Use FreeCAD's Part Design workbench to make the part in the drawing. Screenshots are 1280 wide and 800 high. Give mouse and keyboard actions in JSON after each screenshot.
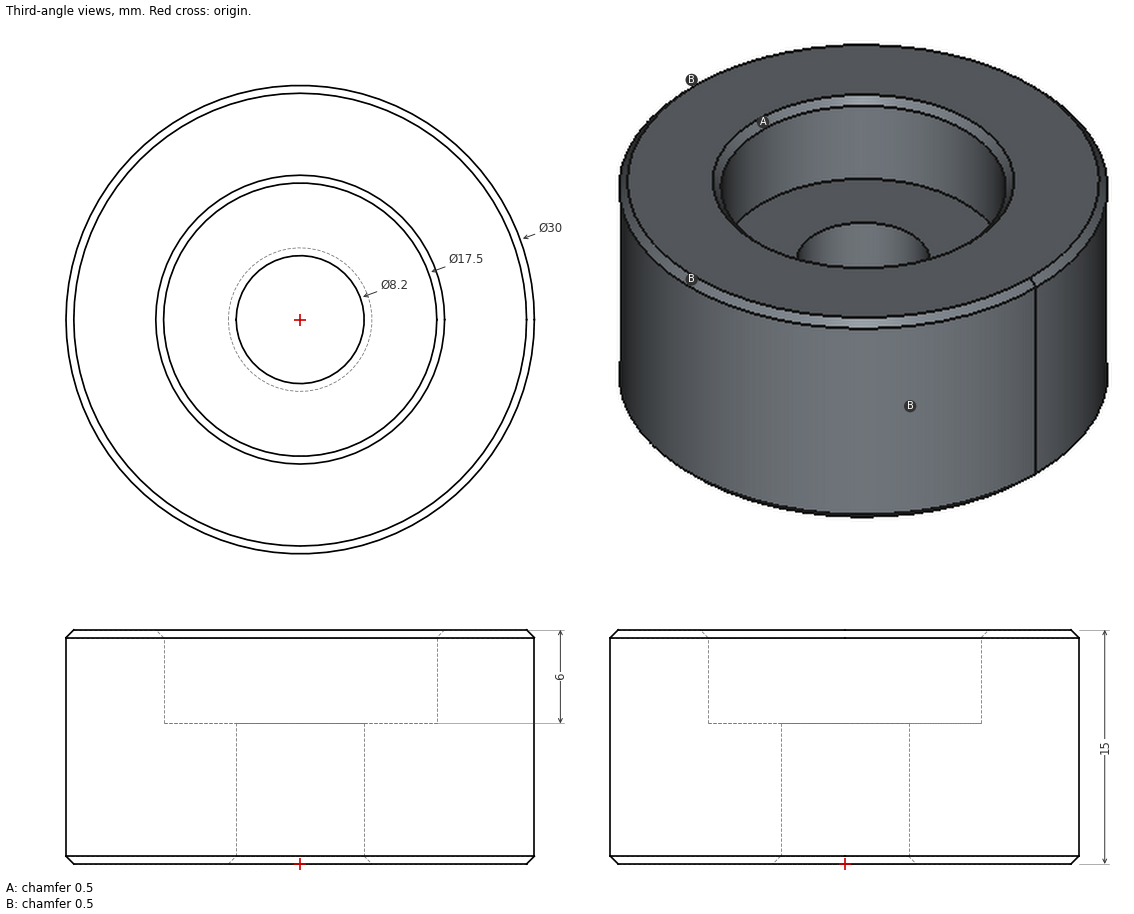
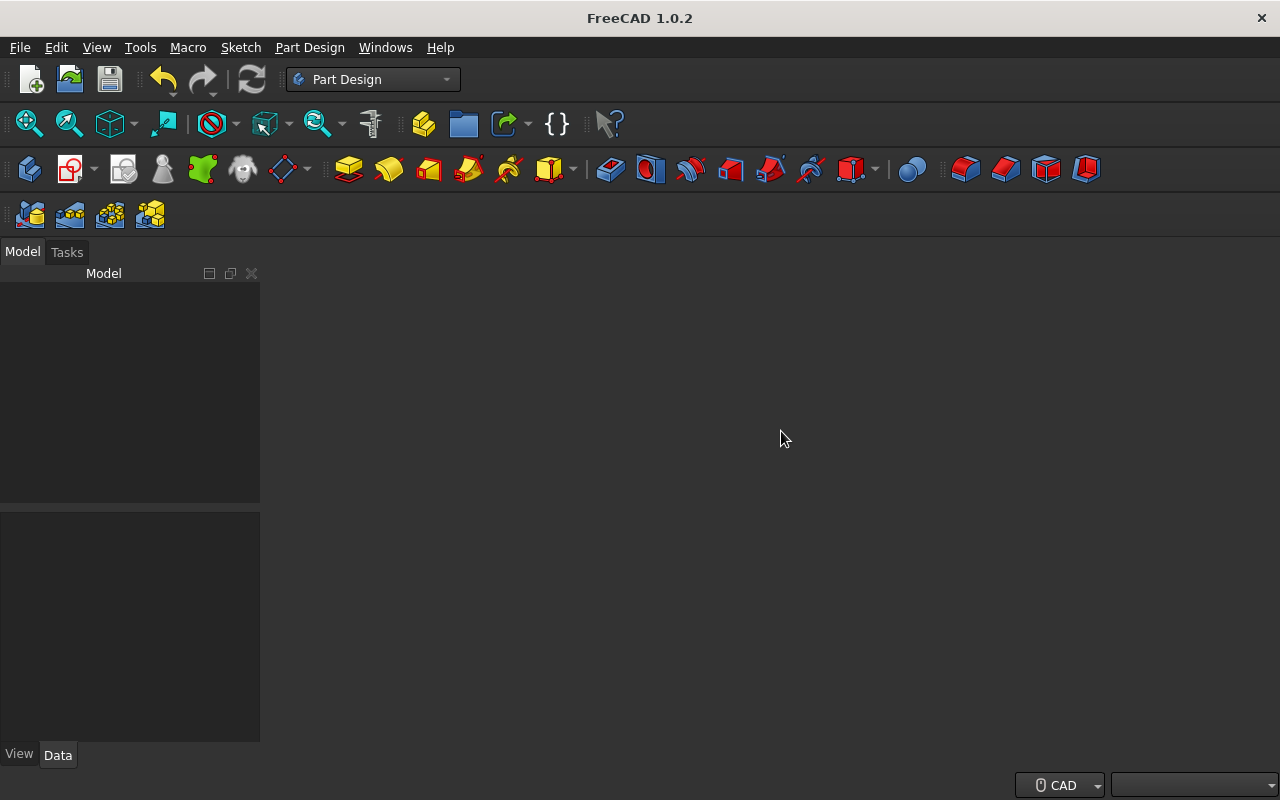
{"action": "key", "text": "ctrl+n"}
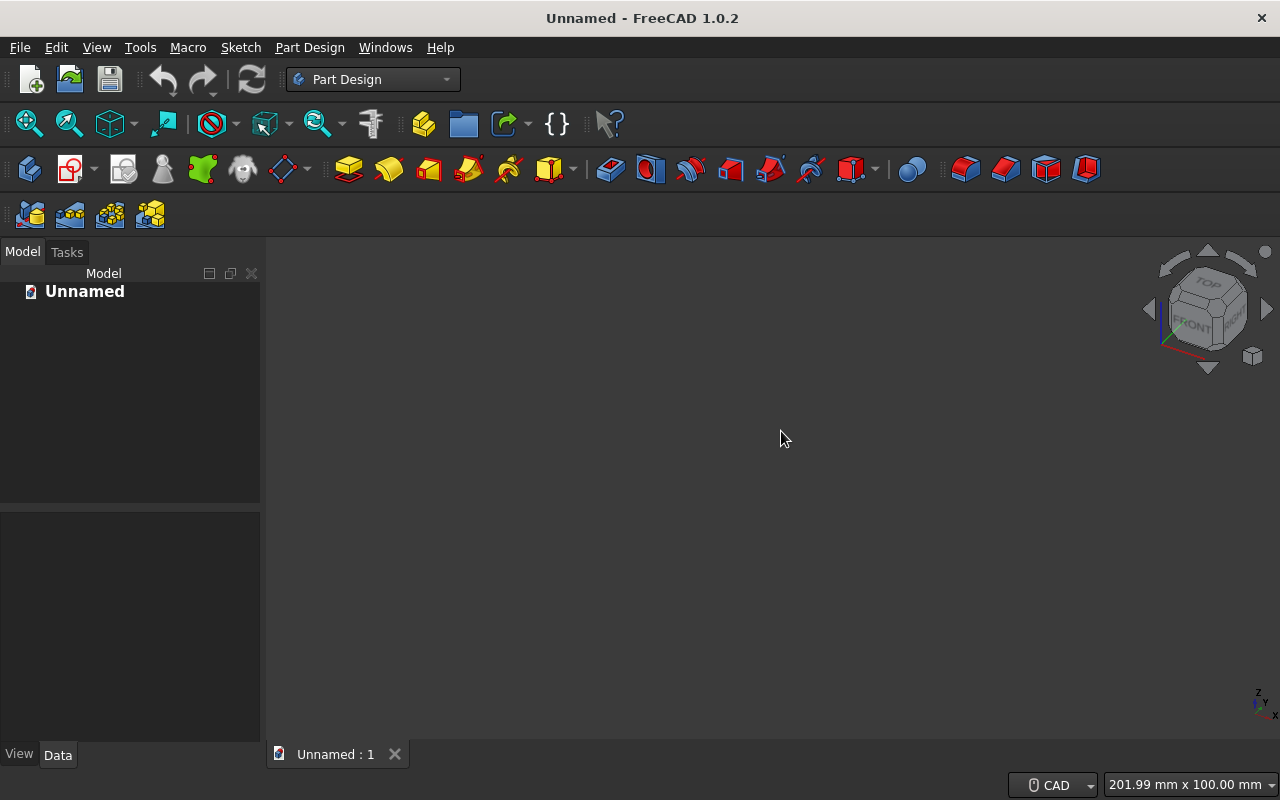
{"action": "left_click", "coordinate": [70, 170]}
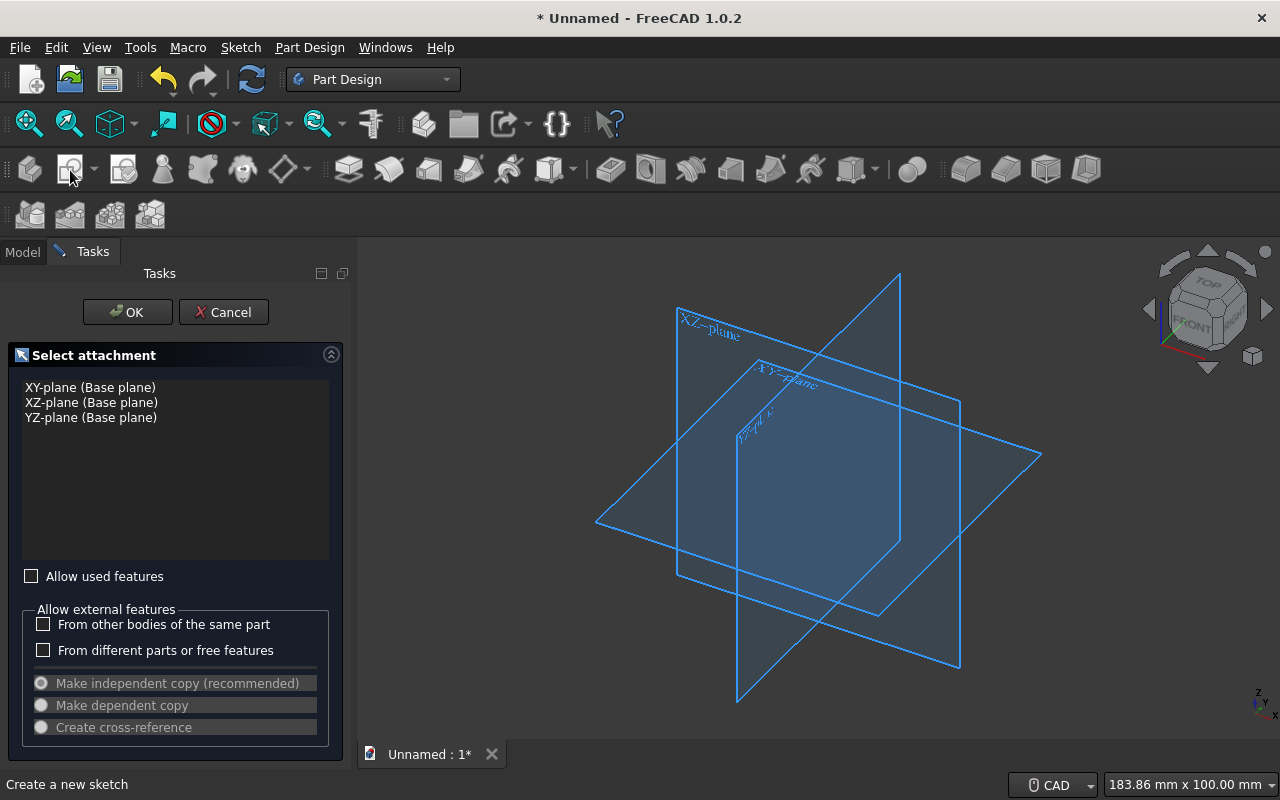
{"action": "left_click", "coordinate": [82, 388]}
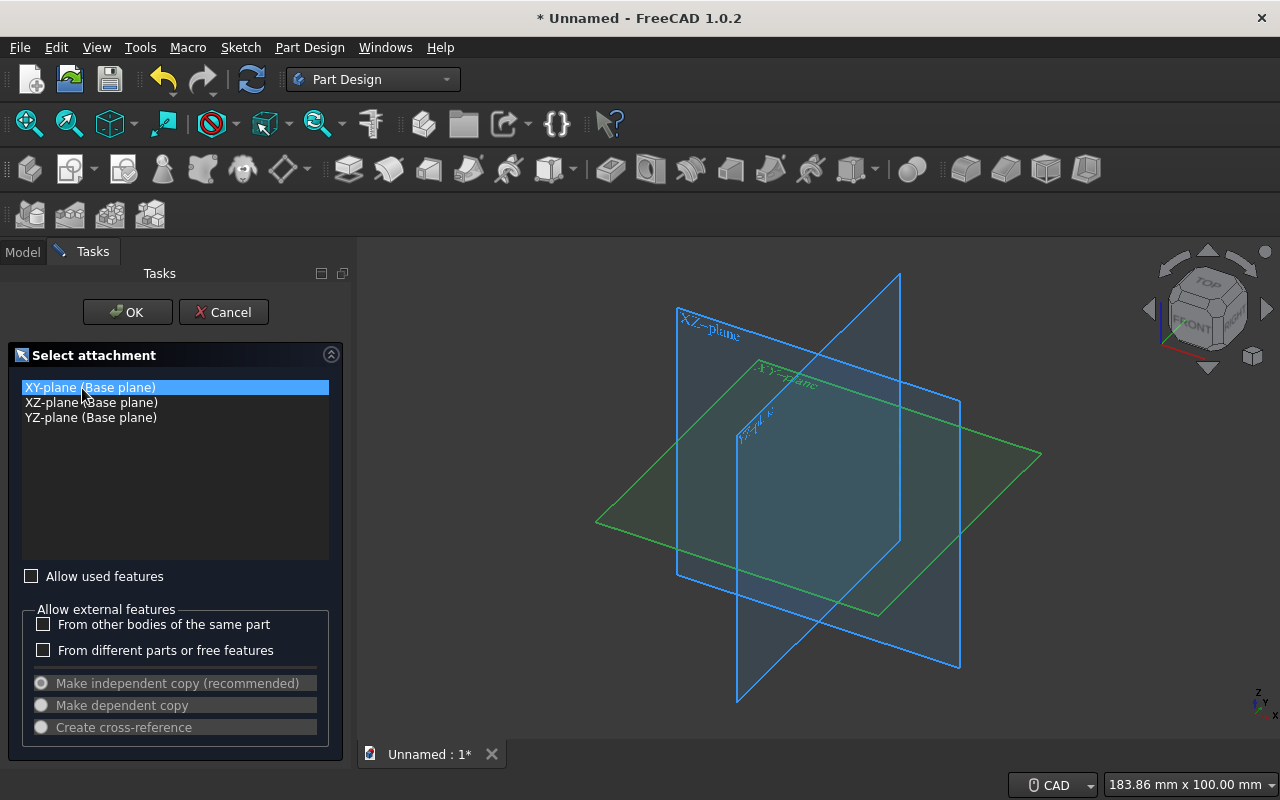
{"action": "left_click", "coordinate": [128, 312]}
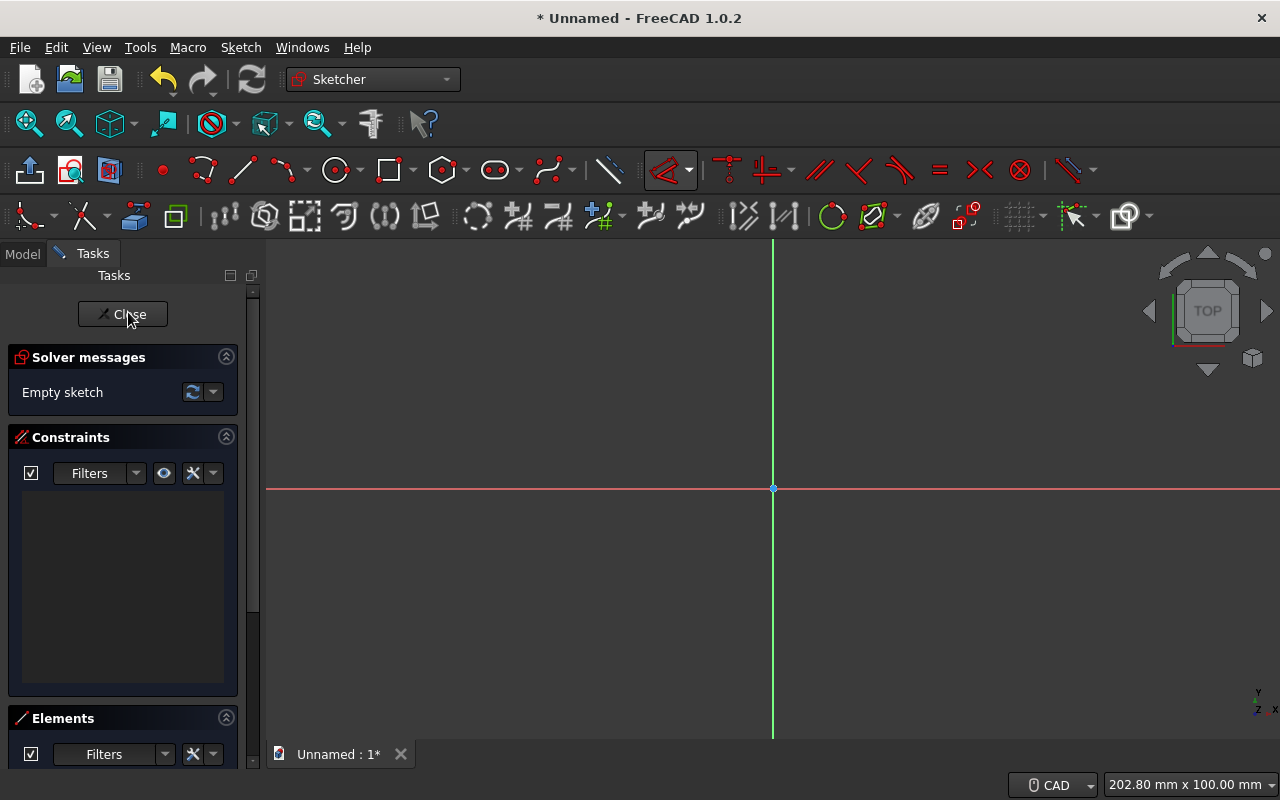
{"action": "scroll", "coordinate": [829, 489], "scroll_direction": "up", "scroll_amount": 4}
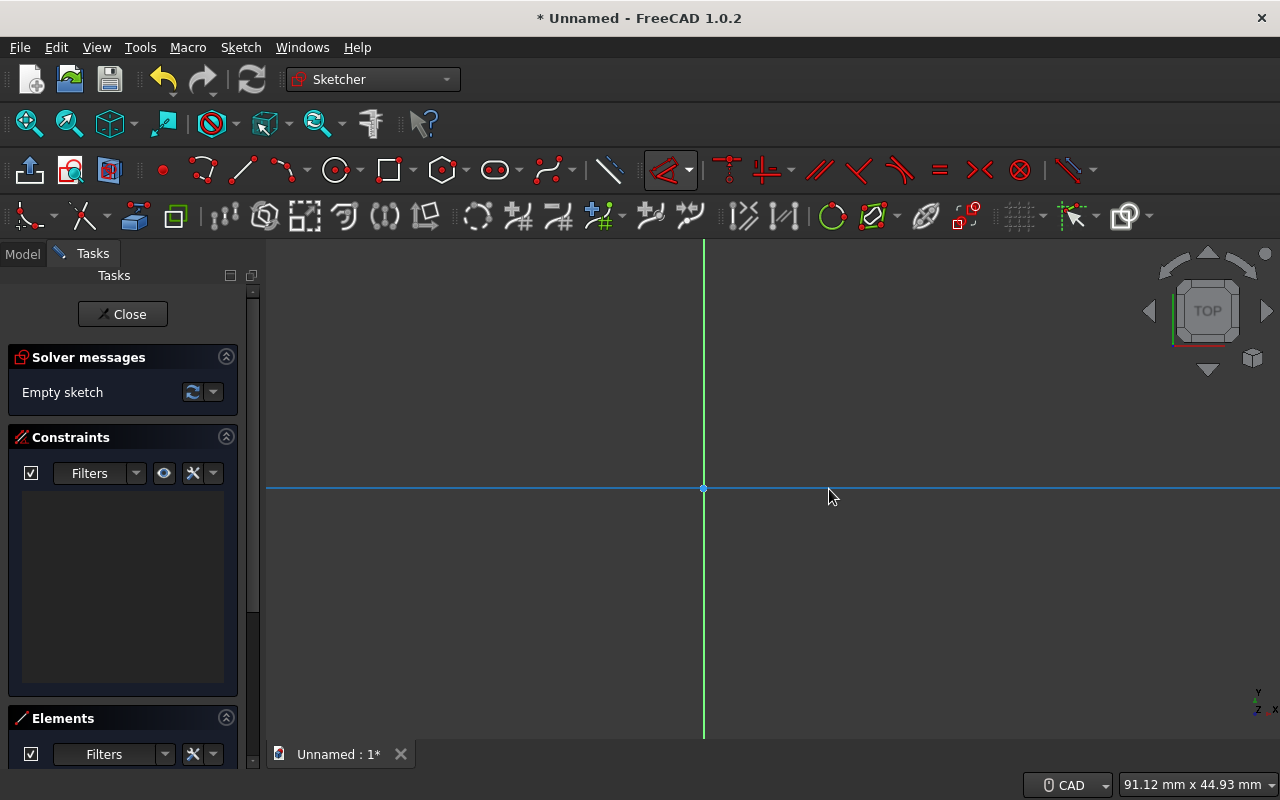
{"action": "left_click", "coordinate": [336, 170]}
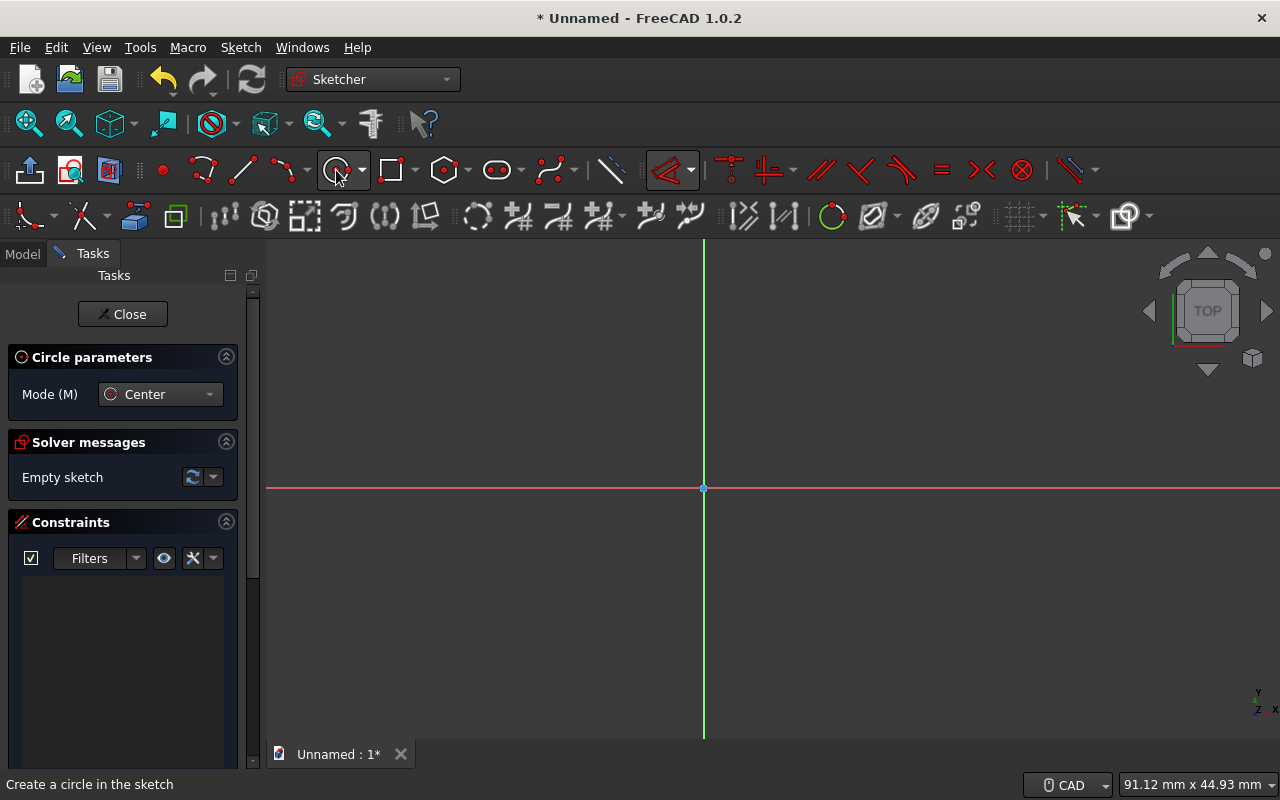
{"action": "left_click", "coordinate": [704, 488]}
{"action": "mouse_move", "coordinate": [822, 370]}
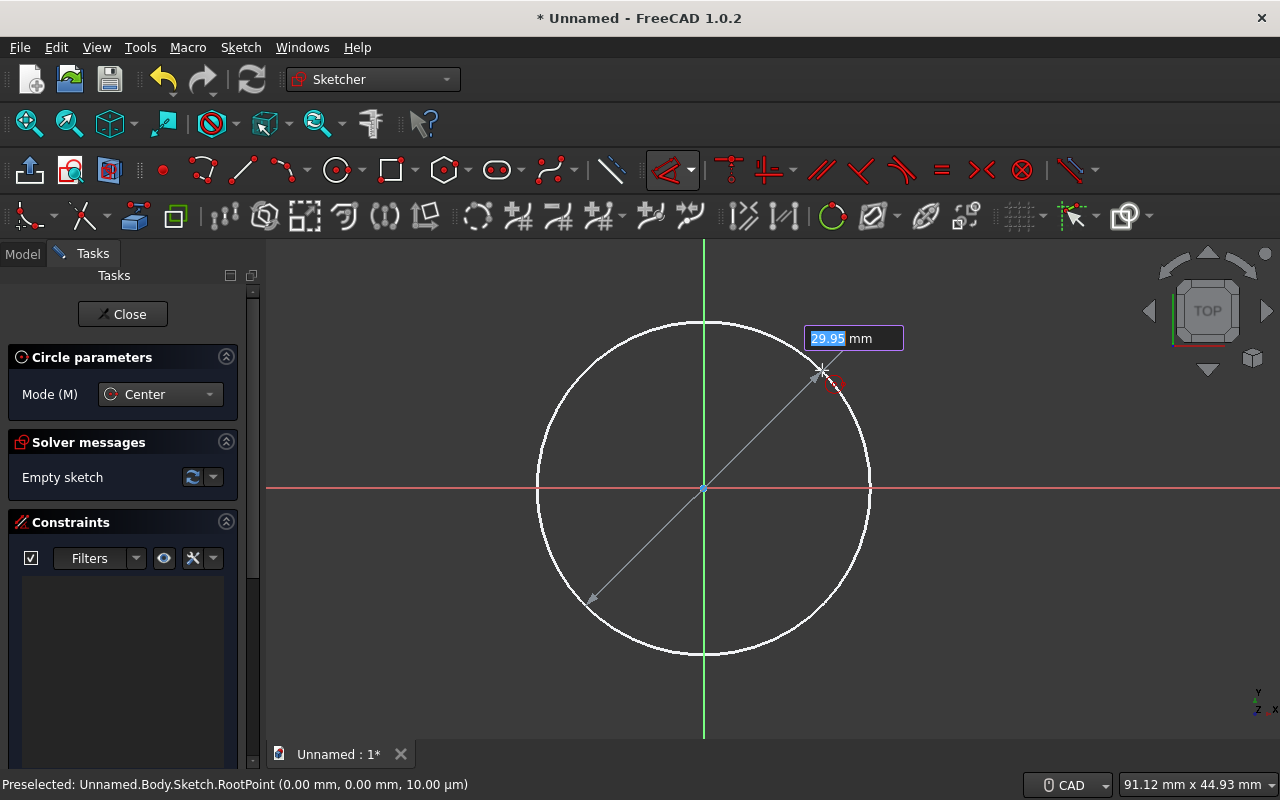
{"action": "type", "text": "30"}
{"action": "key", "text": "Return"}
{"action": "key", "text": "Escape"}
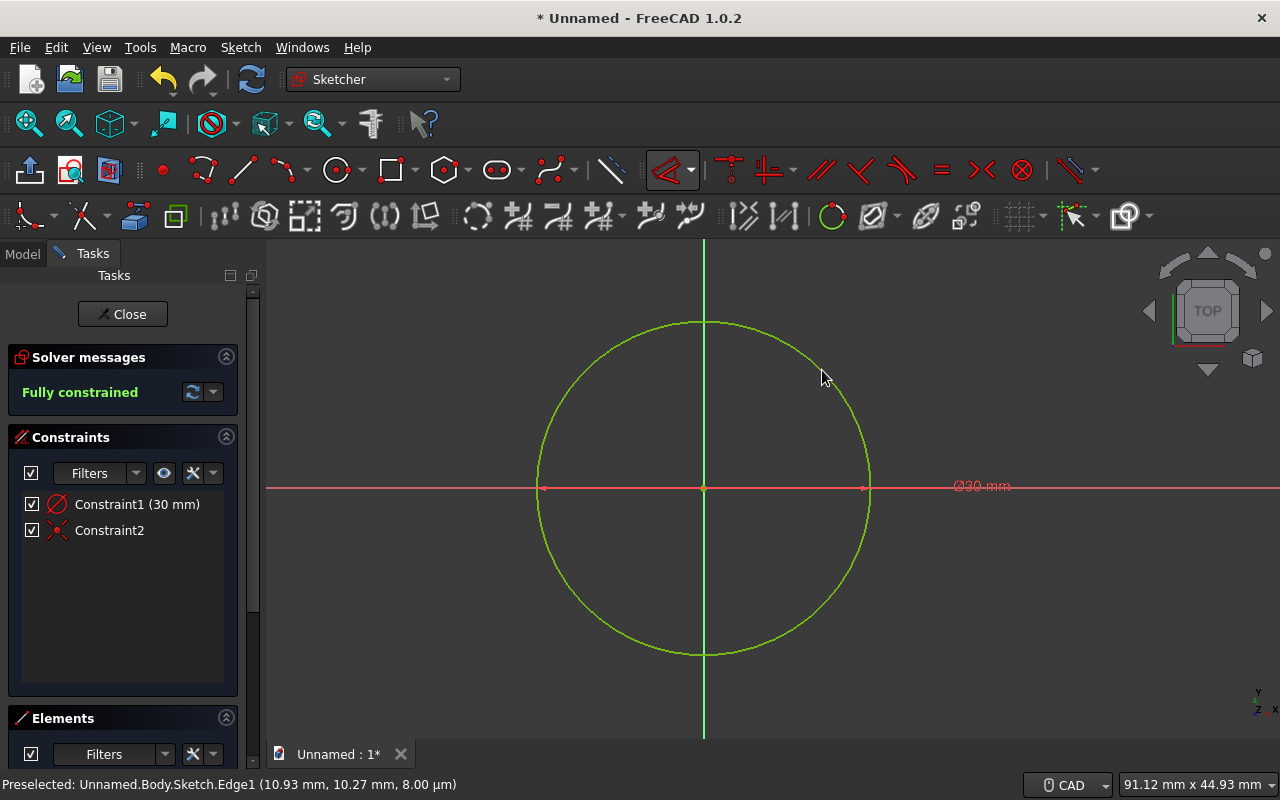
{"action": "left_click", "coordinate": [123, 314]}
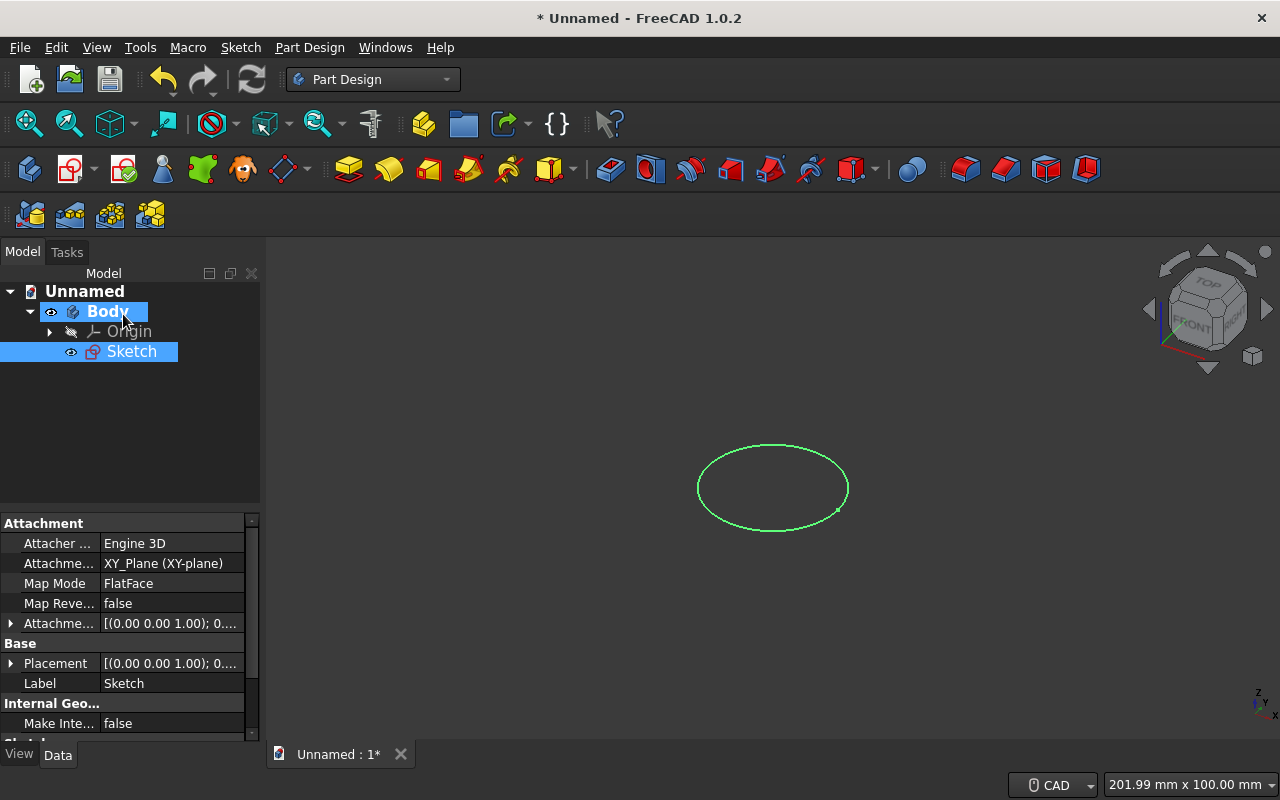
{"action": "left_click", "coordinate": [350, 170]}